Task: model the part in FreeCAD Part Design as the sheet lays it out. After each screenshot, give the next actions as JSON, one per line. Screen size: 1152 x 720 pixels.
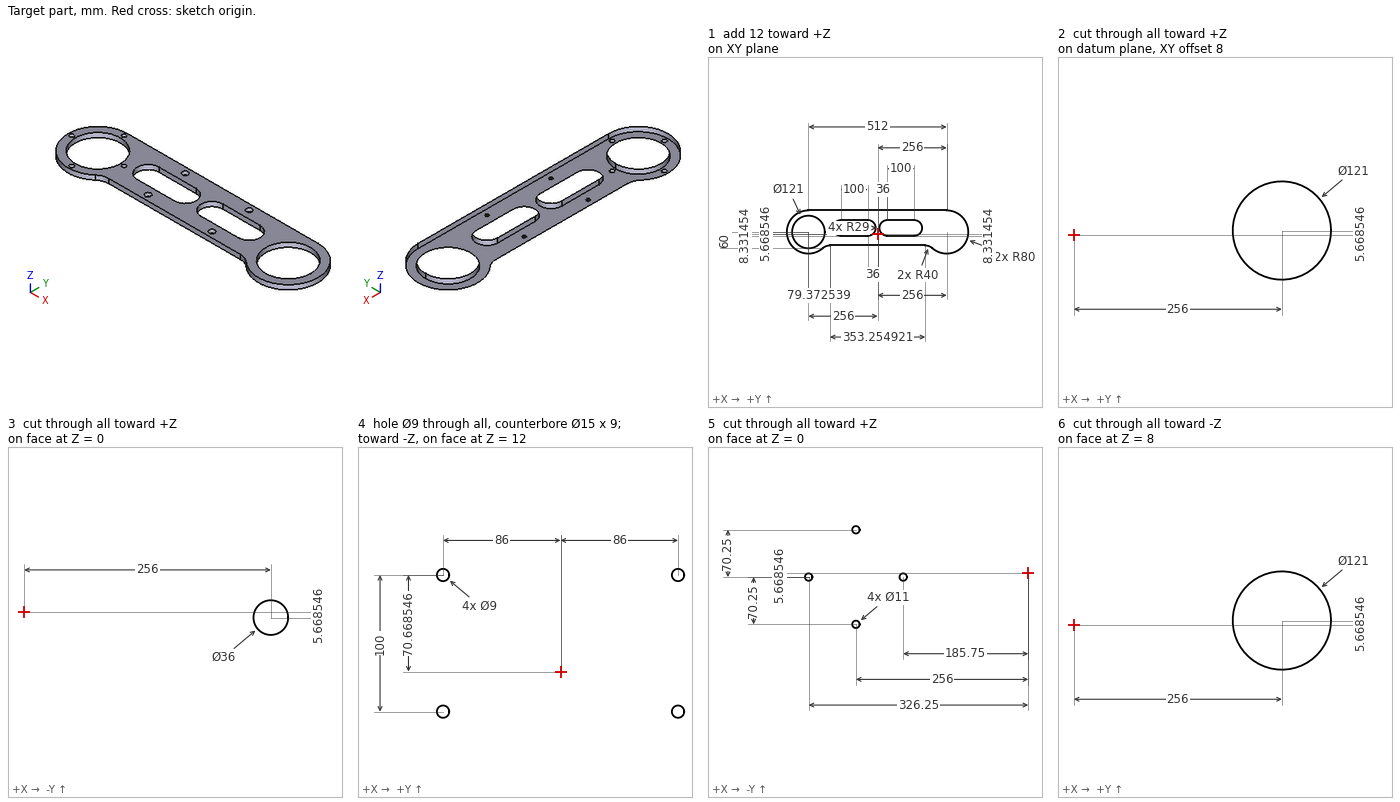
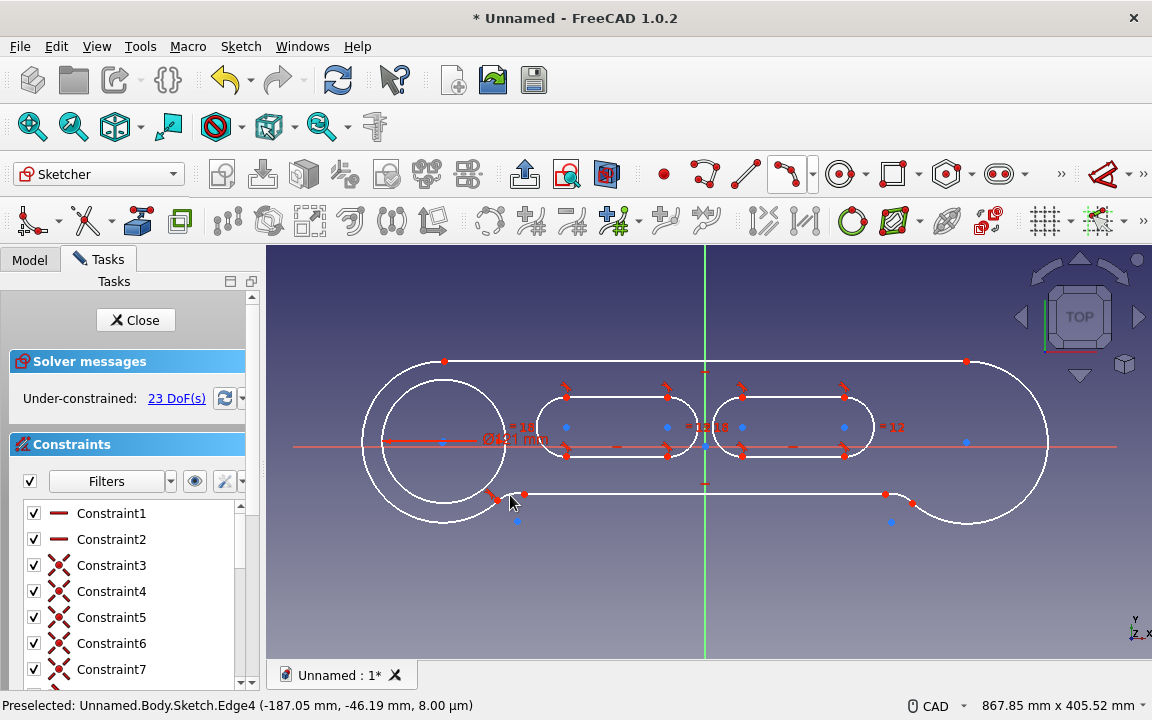
{"action": "left_click", "coordinate": [900, 495]}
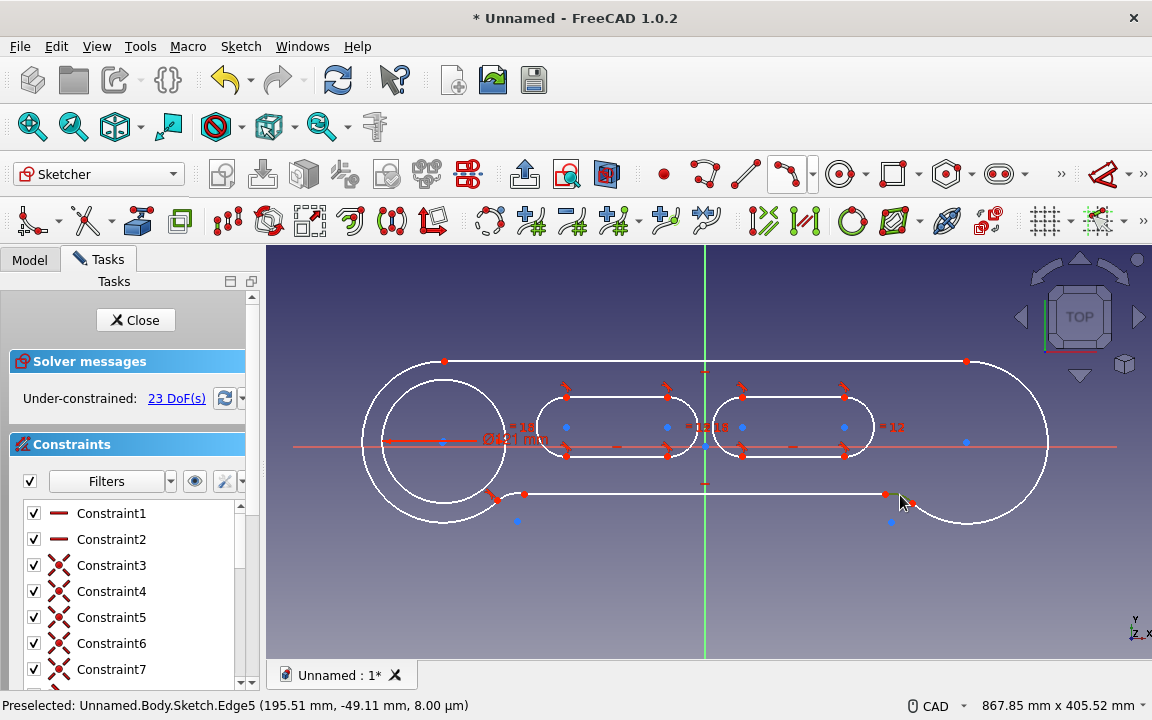
{"action": "left_click", "coordinate": [970, 524]}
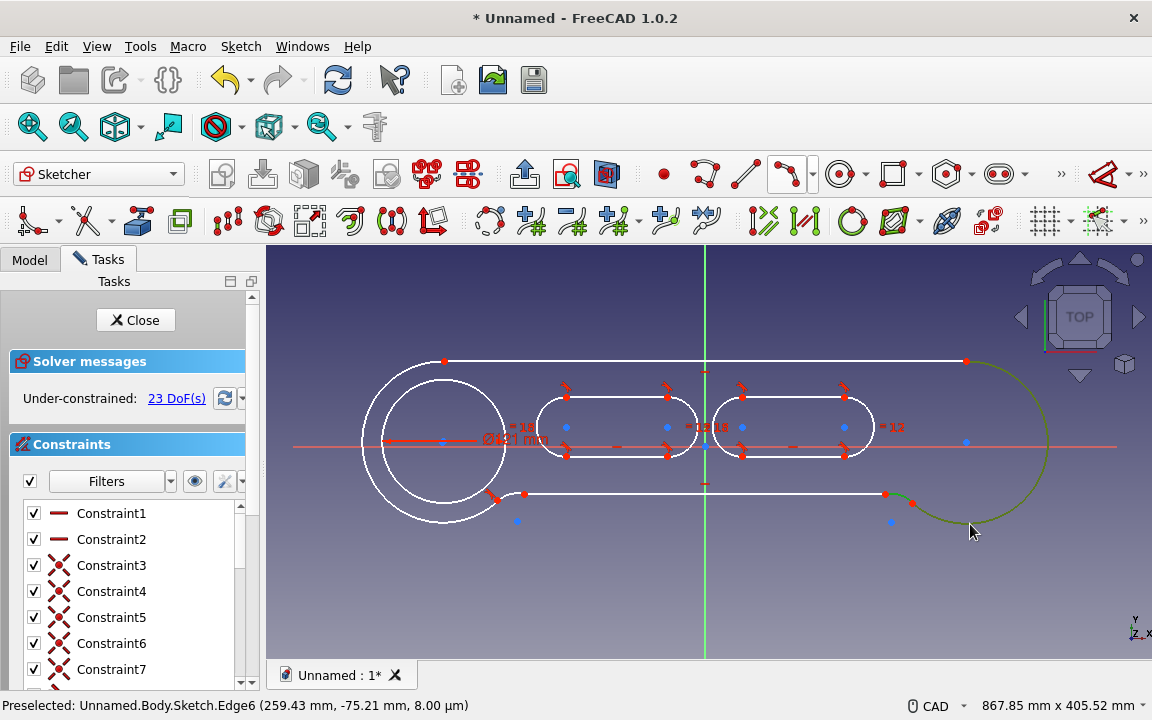
{"action": "key", "text": "t"}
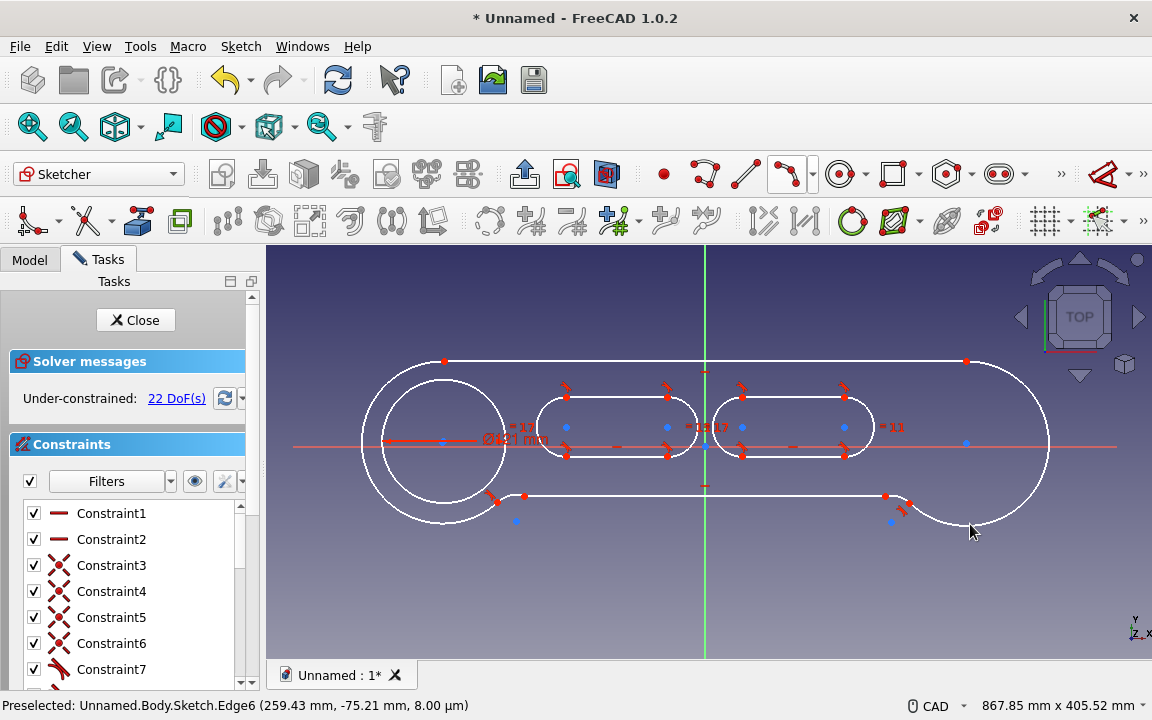
{"action": "left_click", "coordinate": [487, 398]}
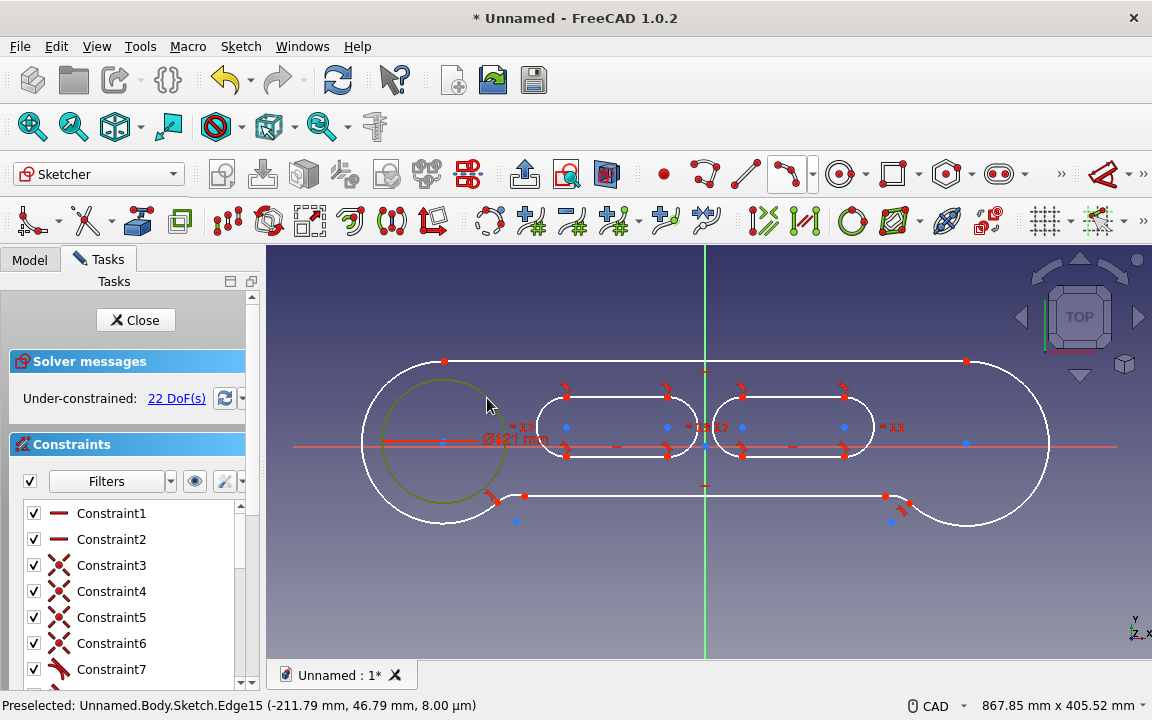
{"action": "left_click", "coordinate": [369, 410]}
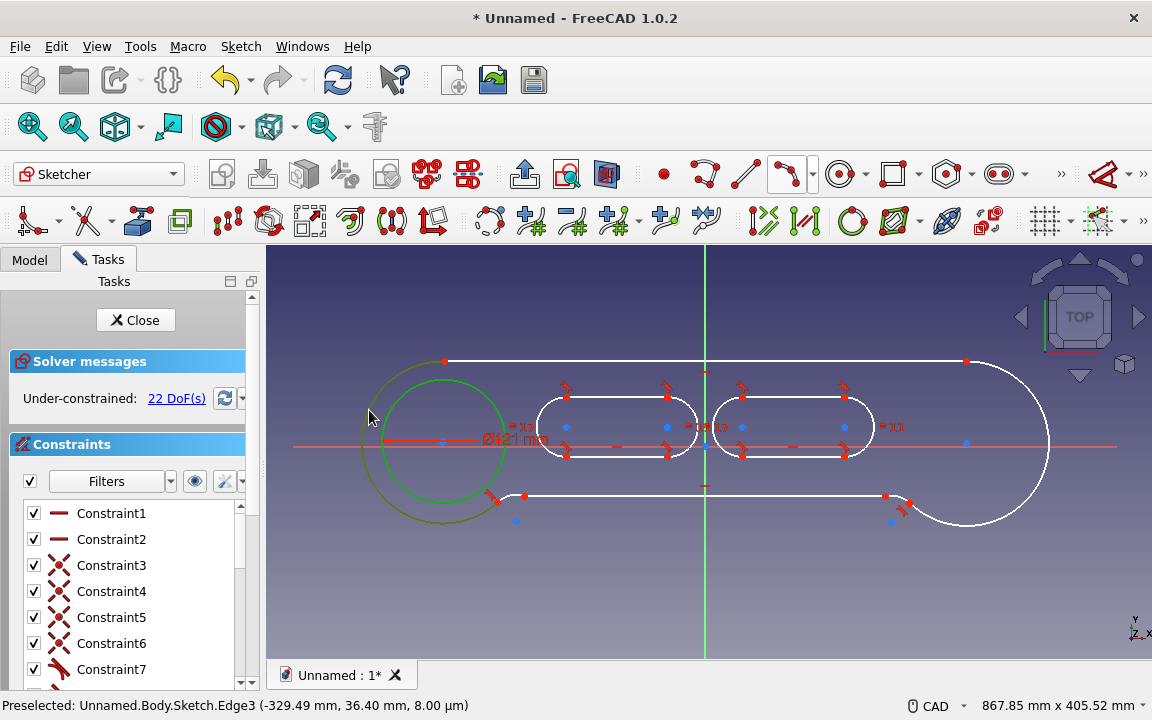
{"action": "key", "text": "c"}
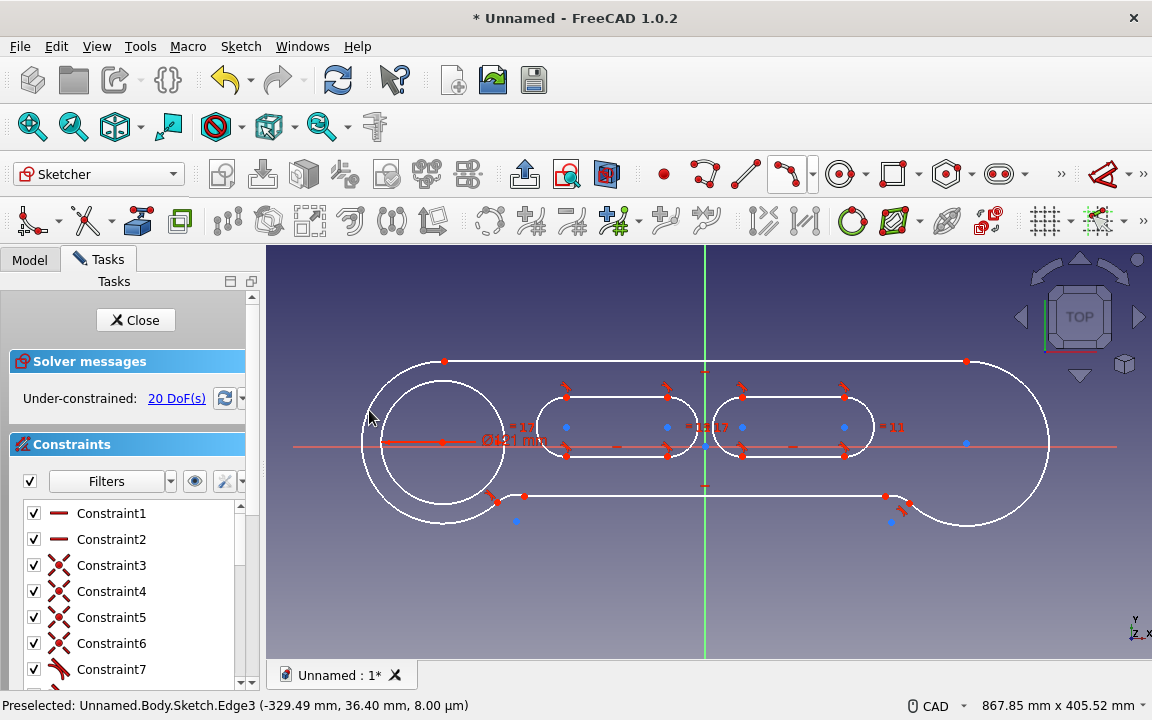
{"action": "left_click", "coordinate": [511, 495]}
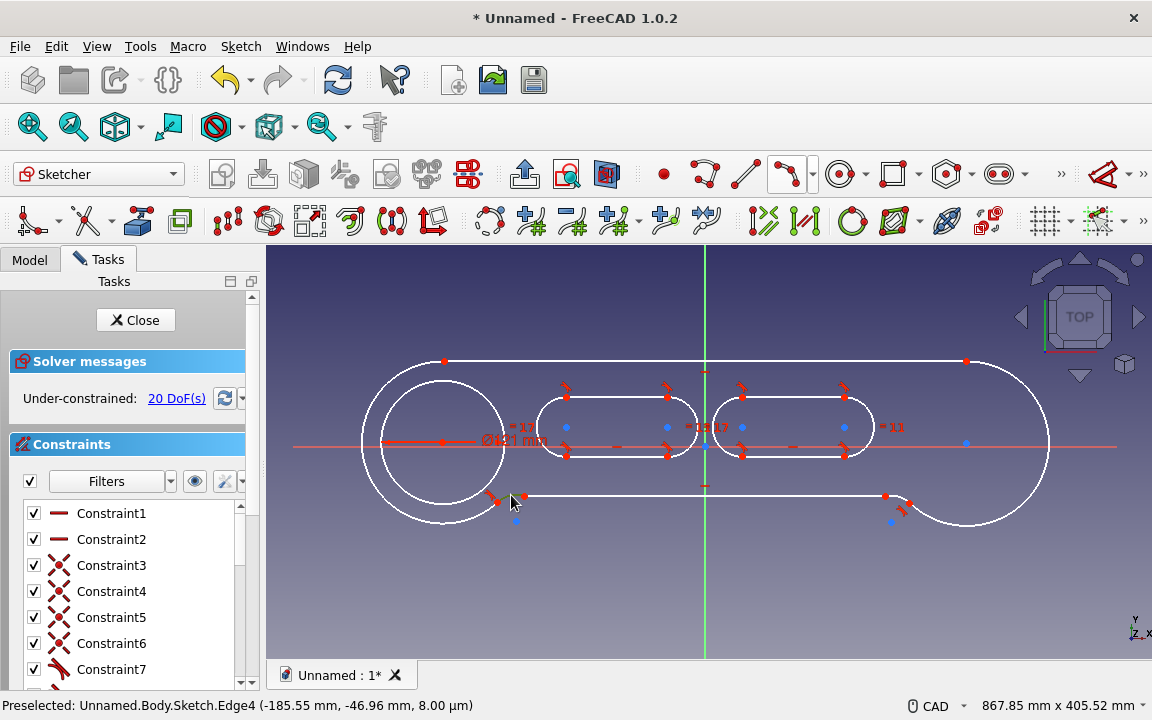
{"action": "left_click", "coordinate": [899, 497]}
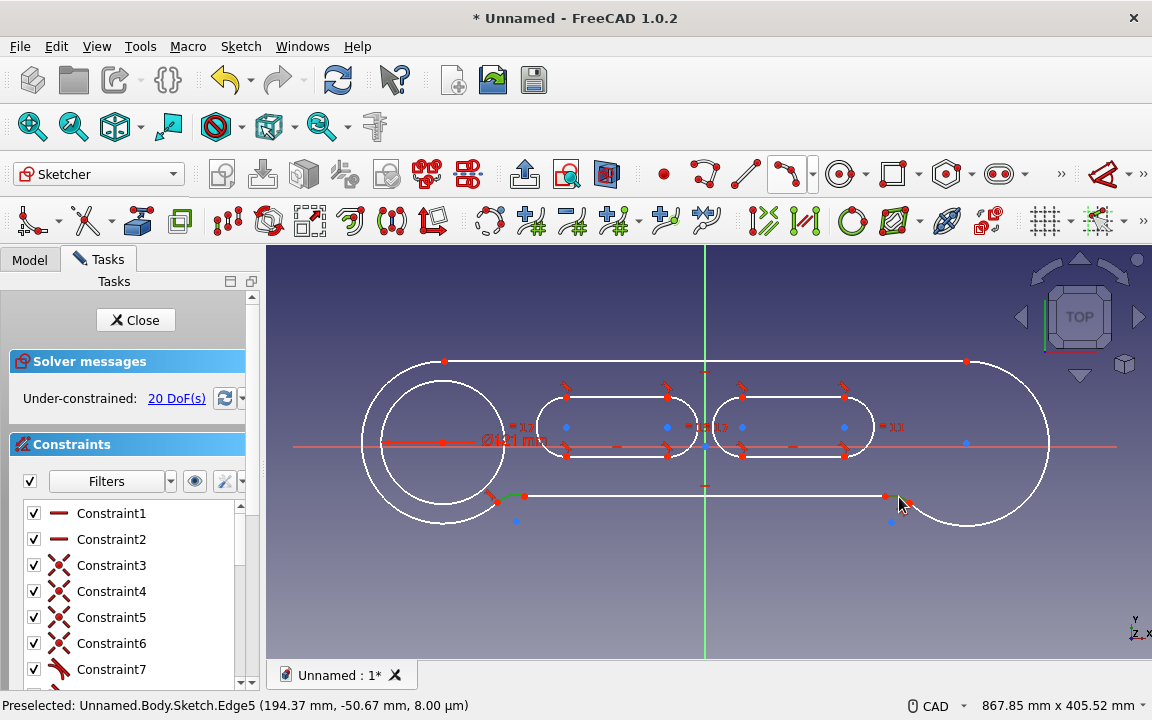
{"action": "key", "text": "e"}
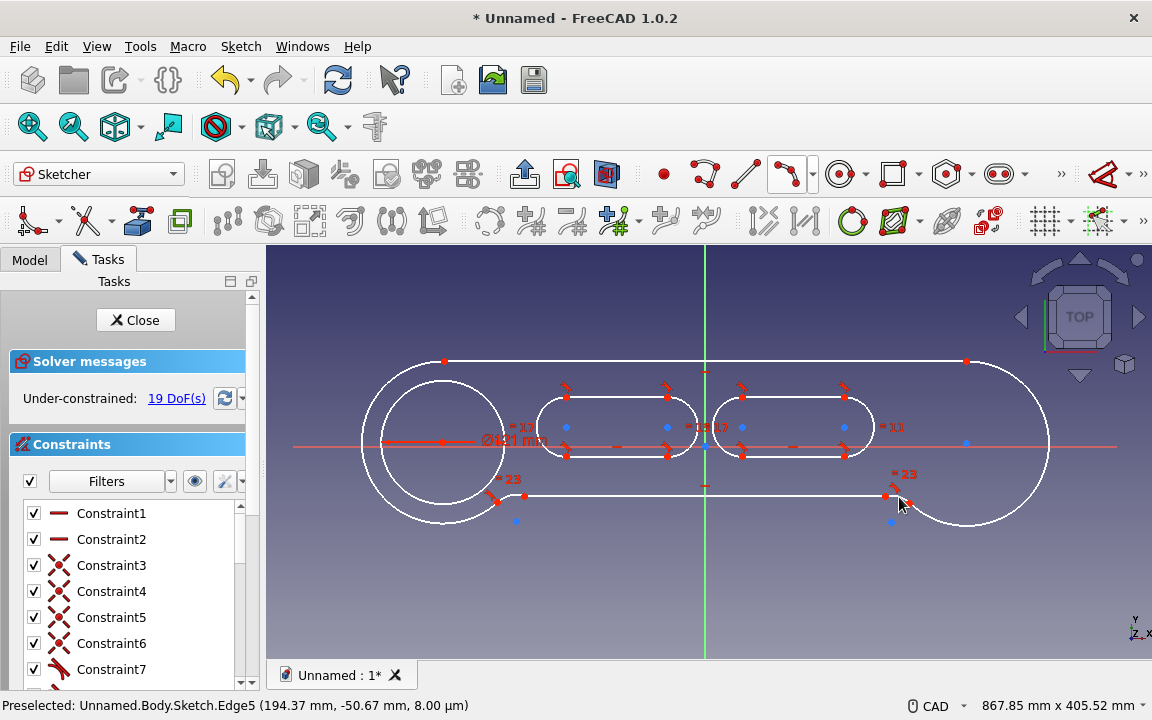
{"action": "left_click", "coordinate": [369, 410]}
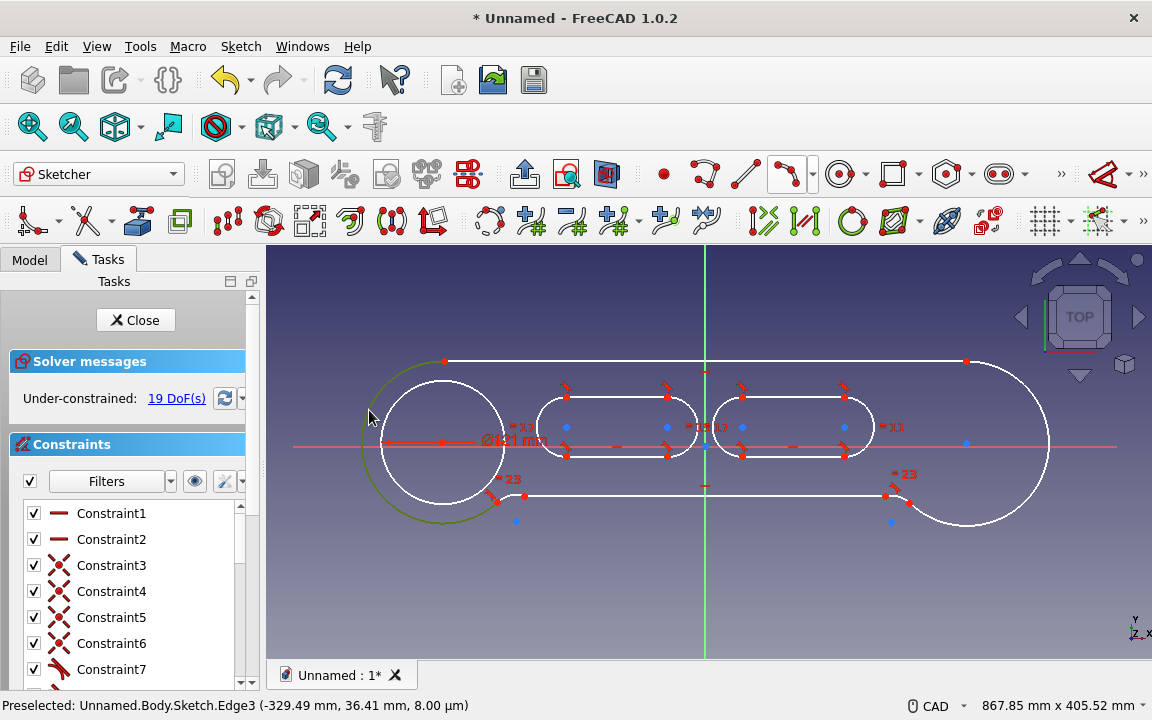
{"action": "left_click", "coordinate": [968, 526]}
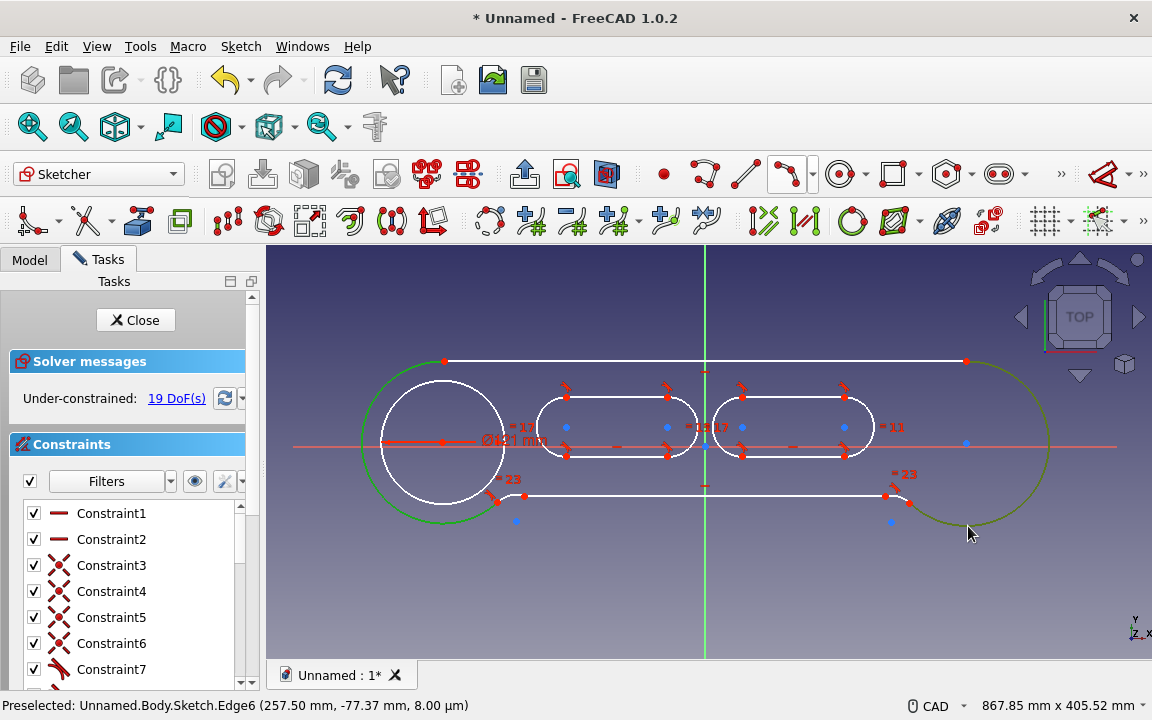
{"action": "key", "text": "e"}